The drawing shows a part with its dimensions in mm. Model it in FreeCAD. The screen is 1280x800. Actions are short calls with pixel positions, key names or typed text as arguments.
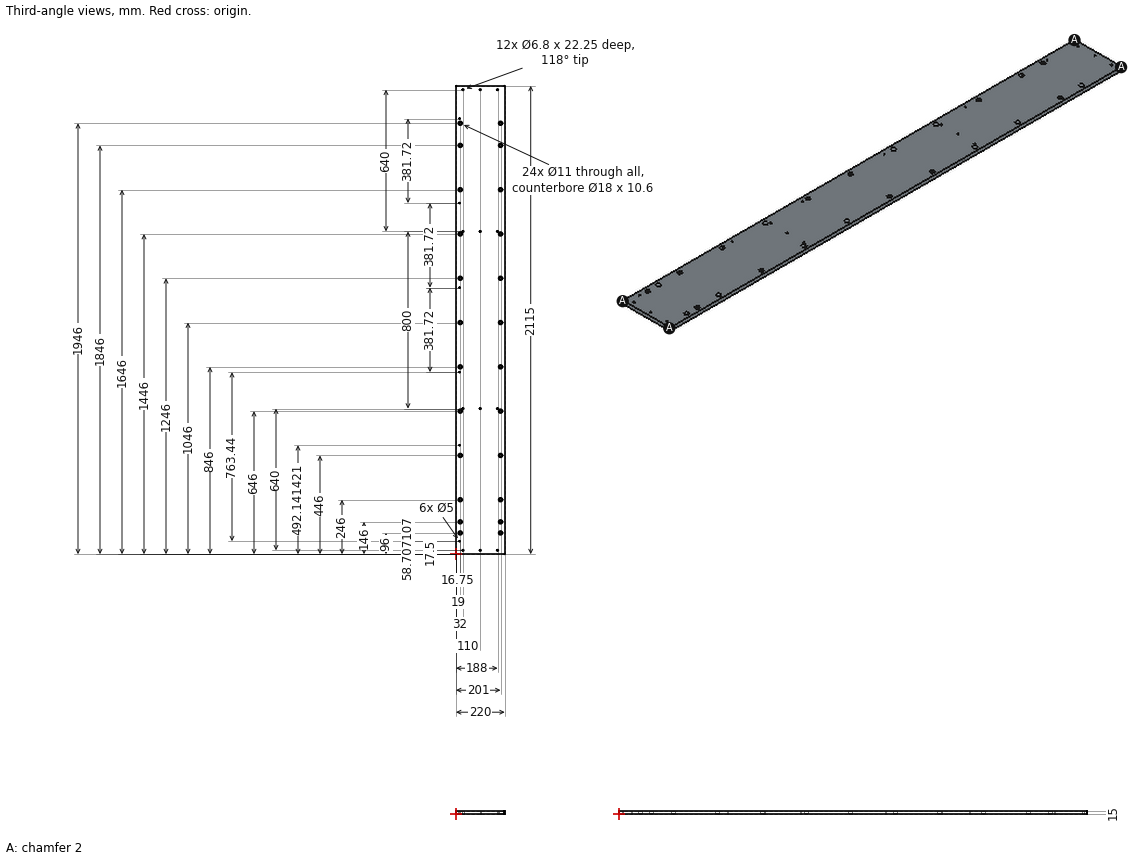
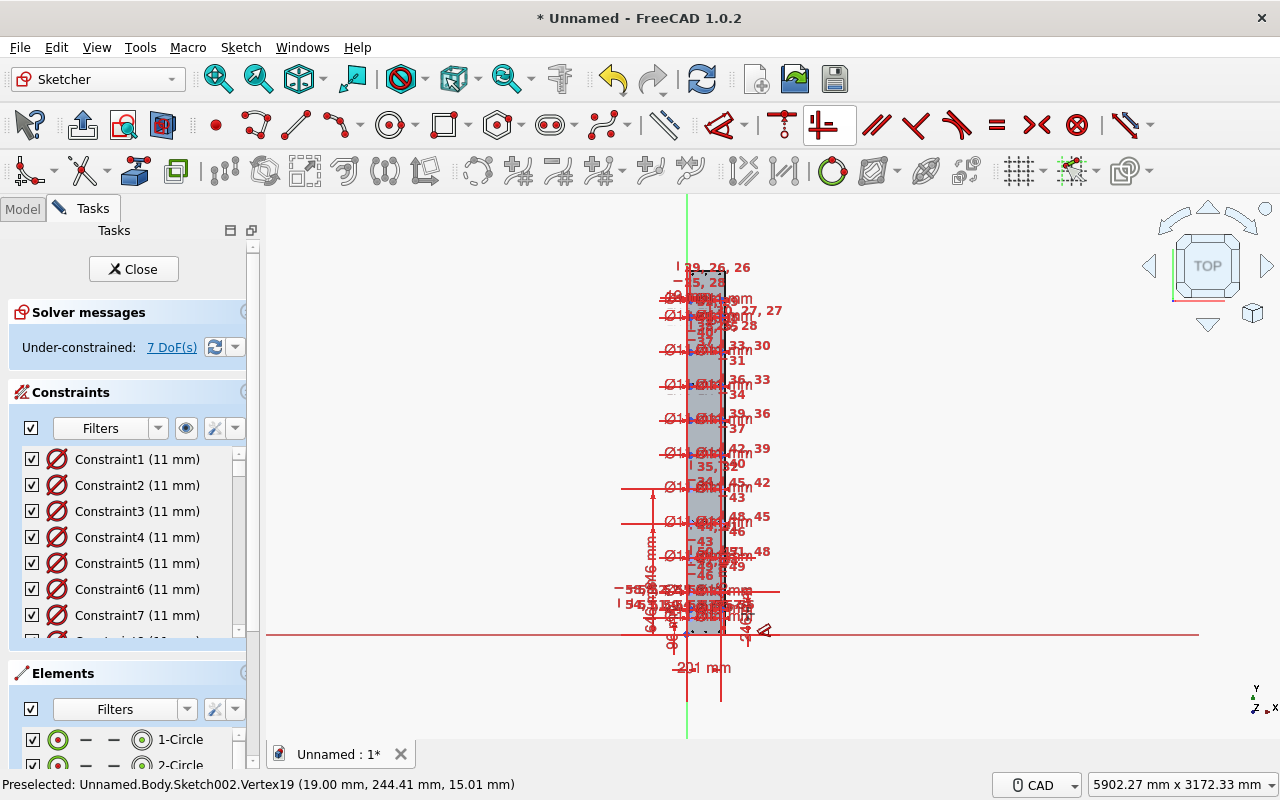
scroll(690, 610, up, 3)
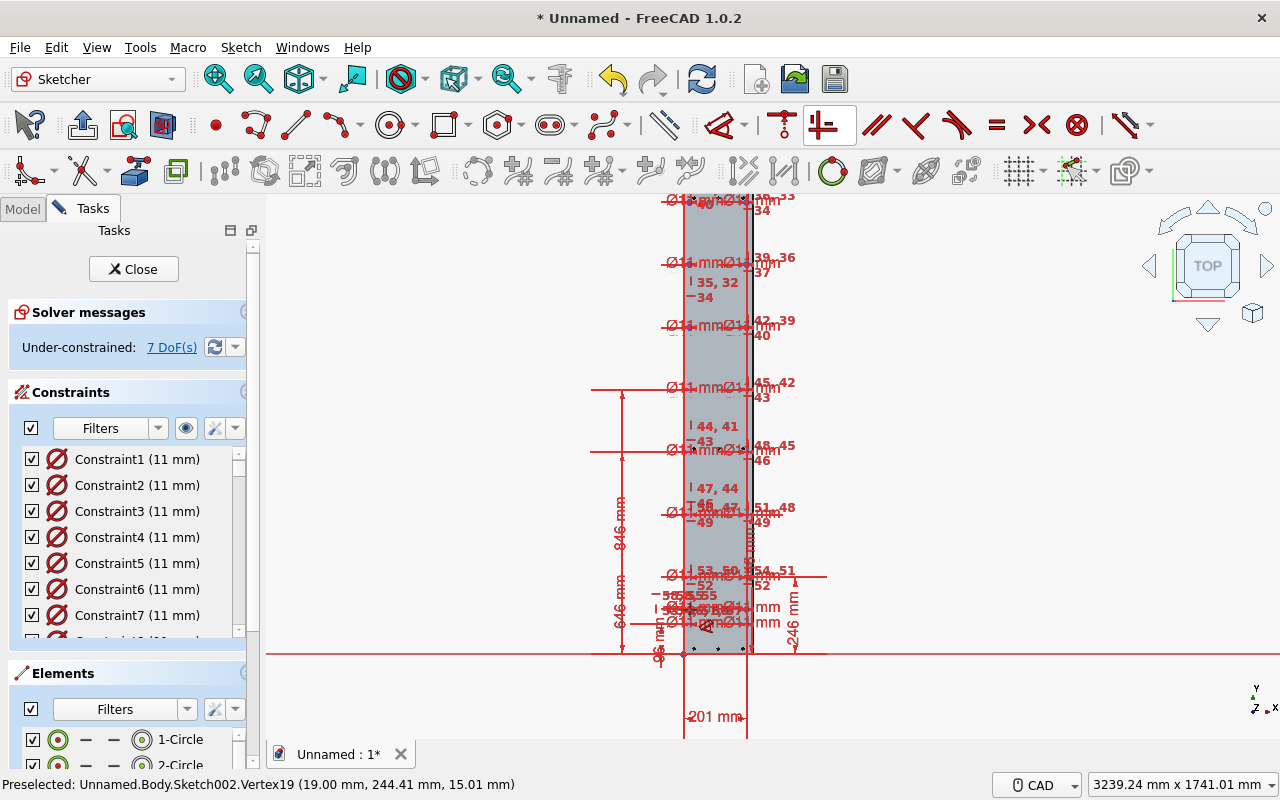
click(690, 609)
click(724, 616)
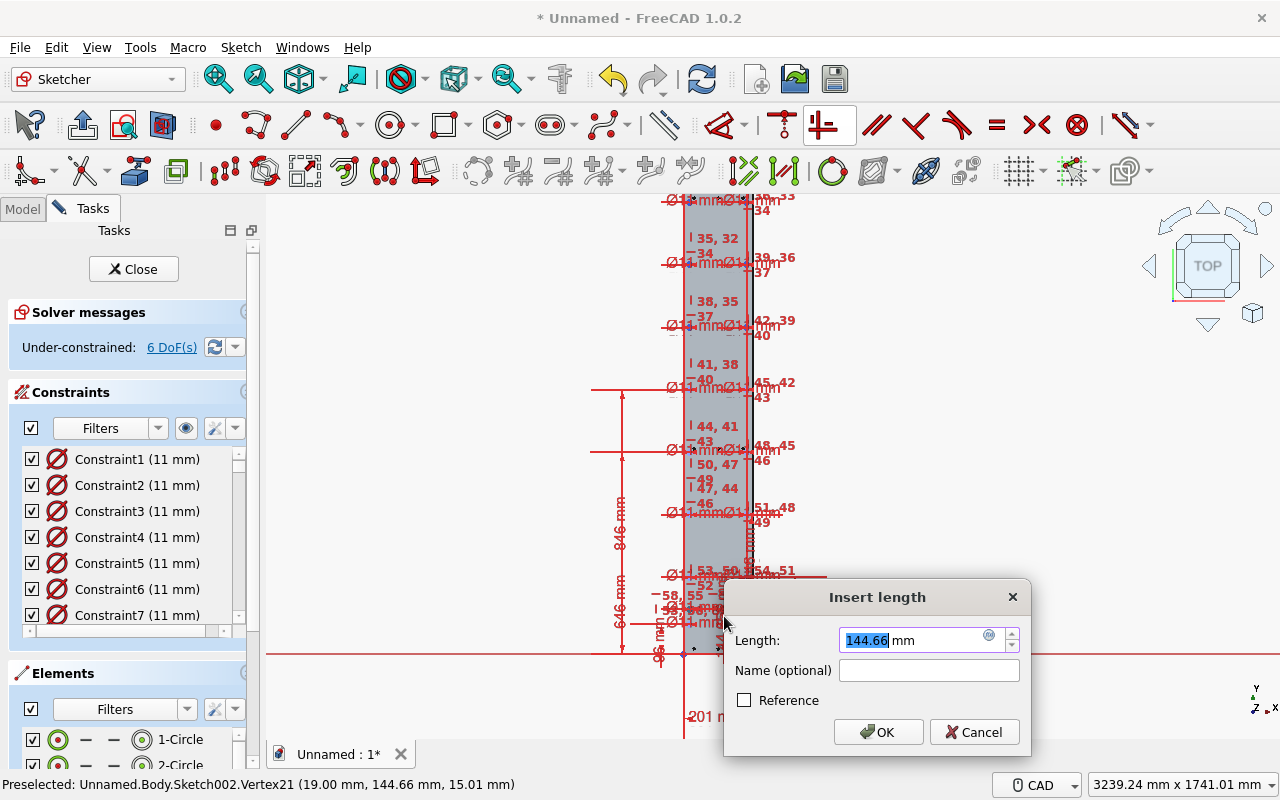
text(146)
key(Return)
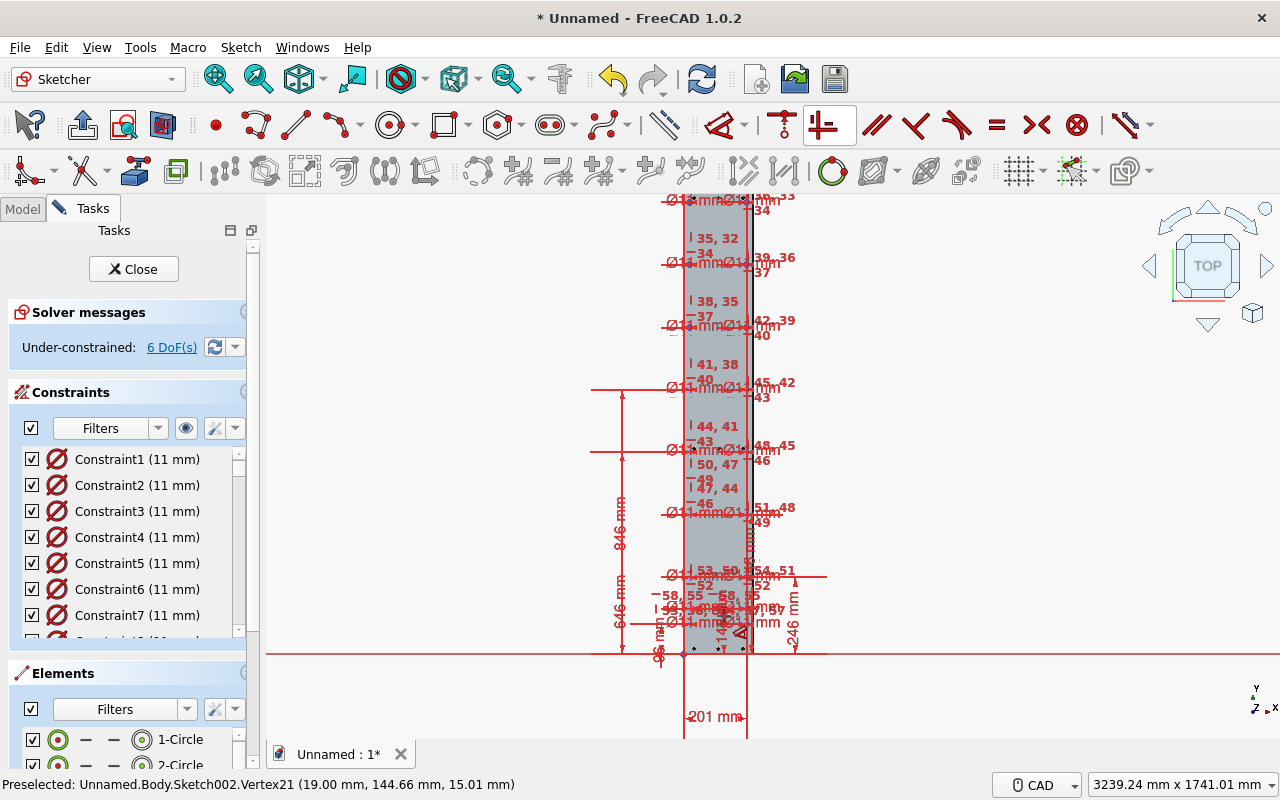
scroll(690, 609, down, 3)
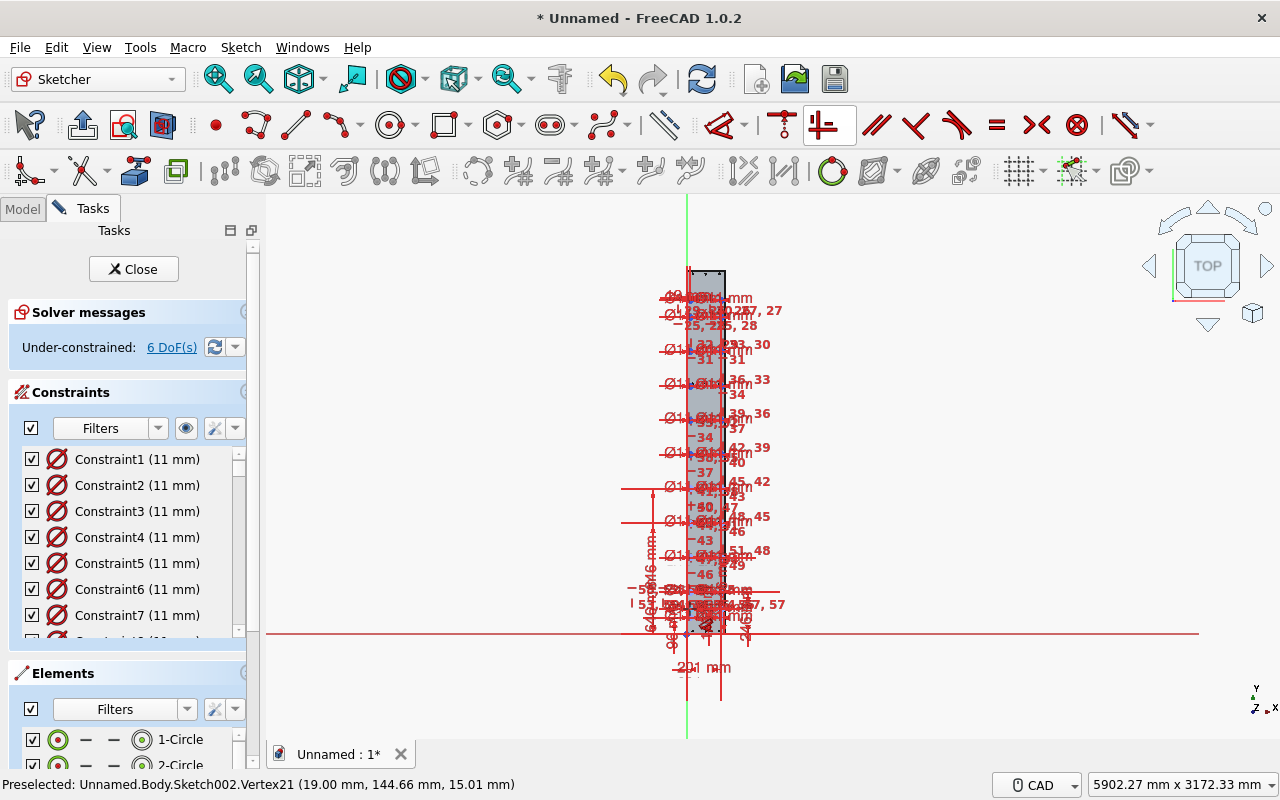
click(690, 300)
click(653, 467)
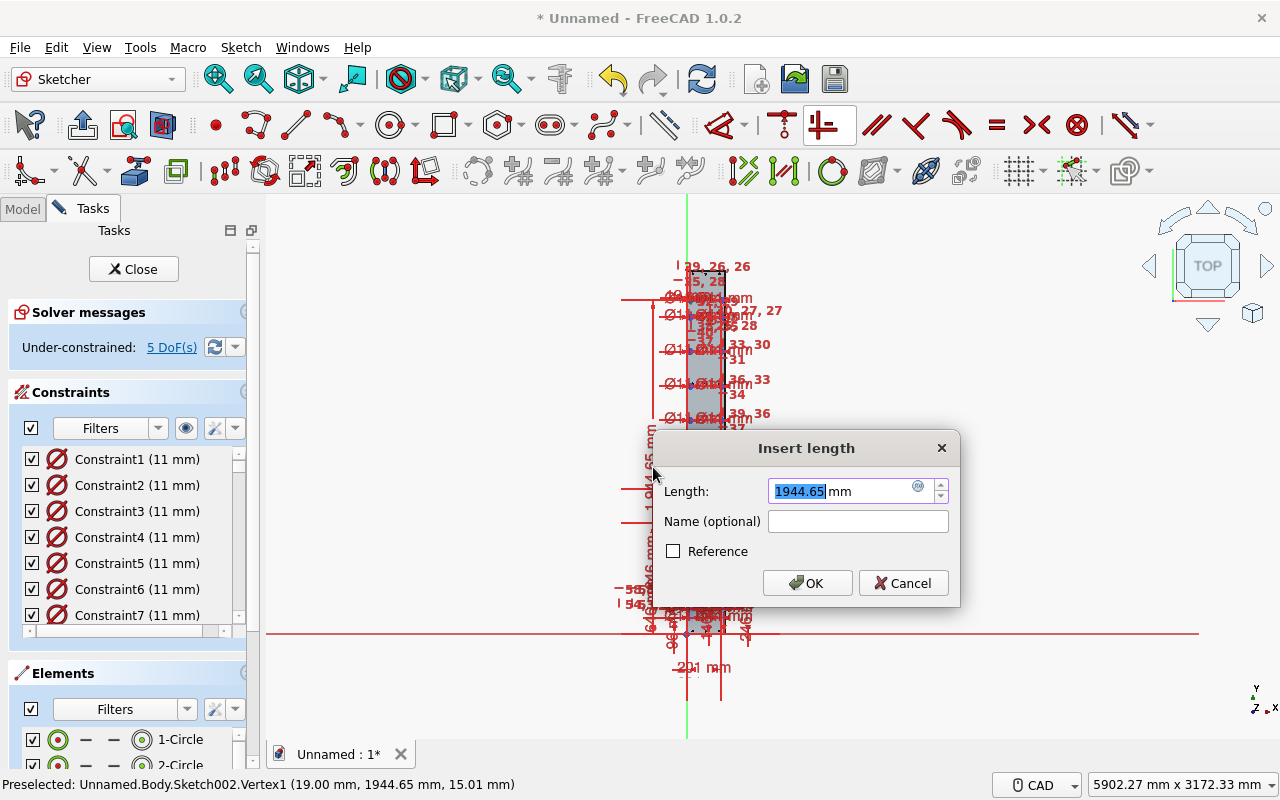
text(1946)
key(Return)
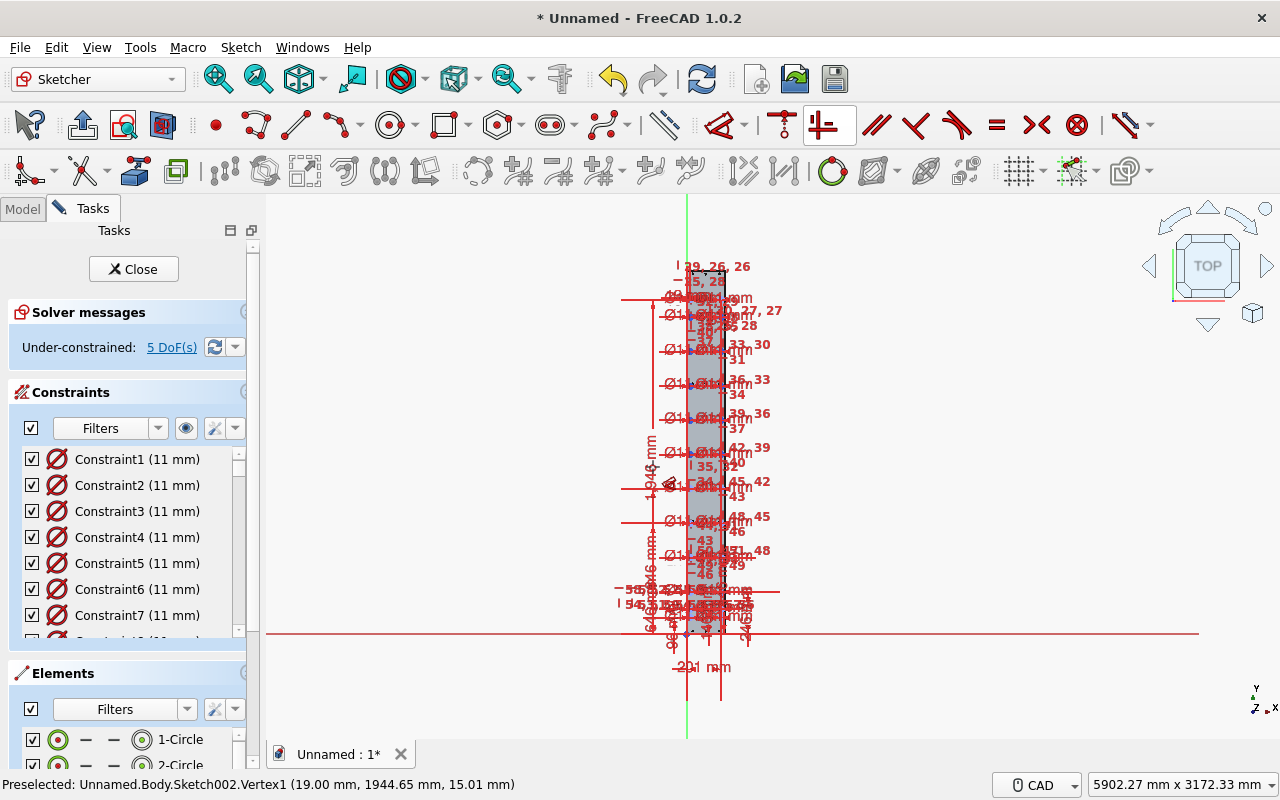
click(690, 317)
click(653, 403)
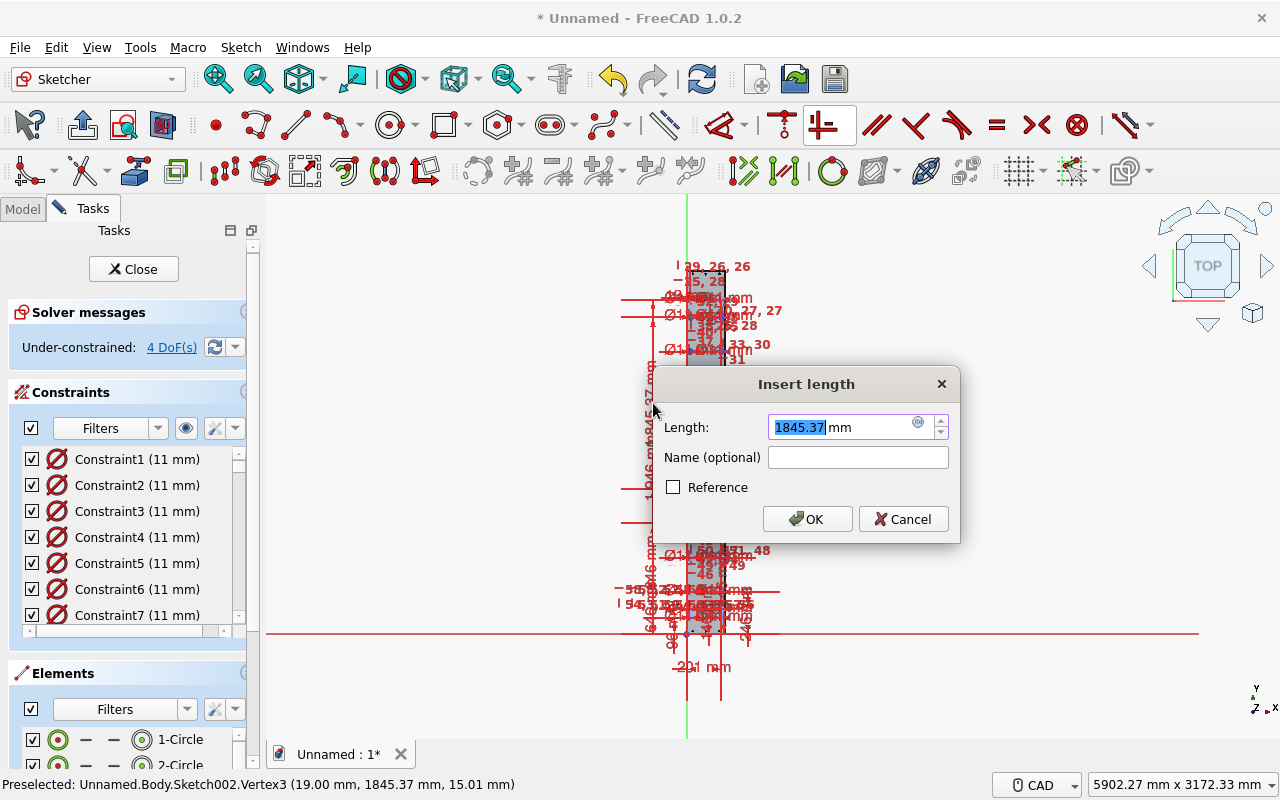
text(1846)
key(Return)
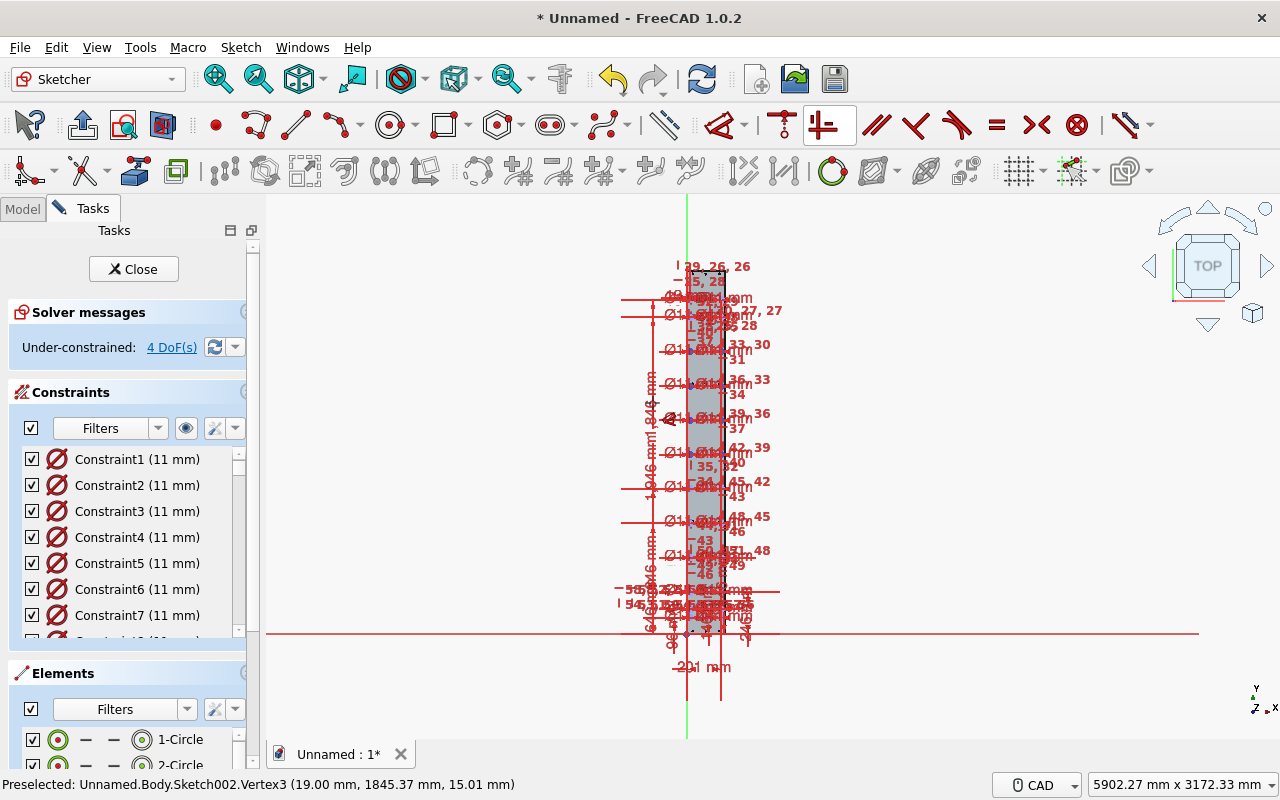
click(690, 352)
click(653, 493)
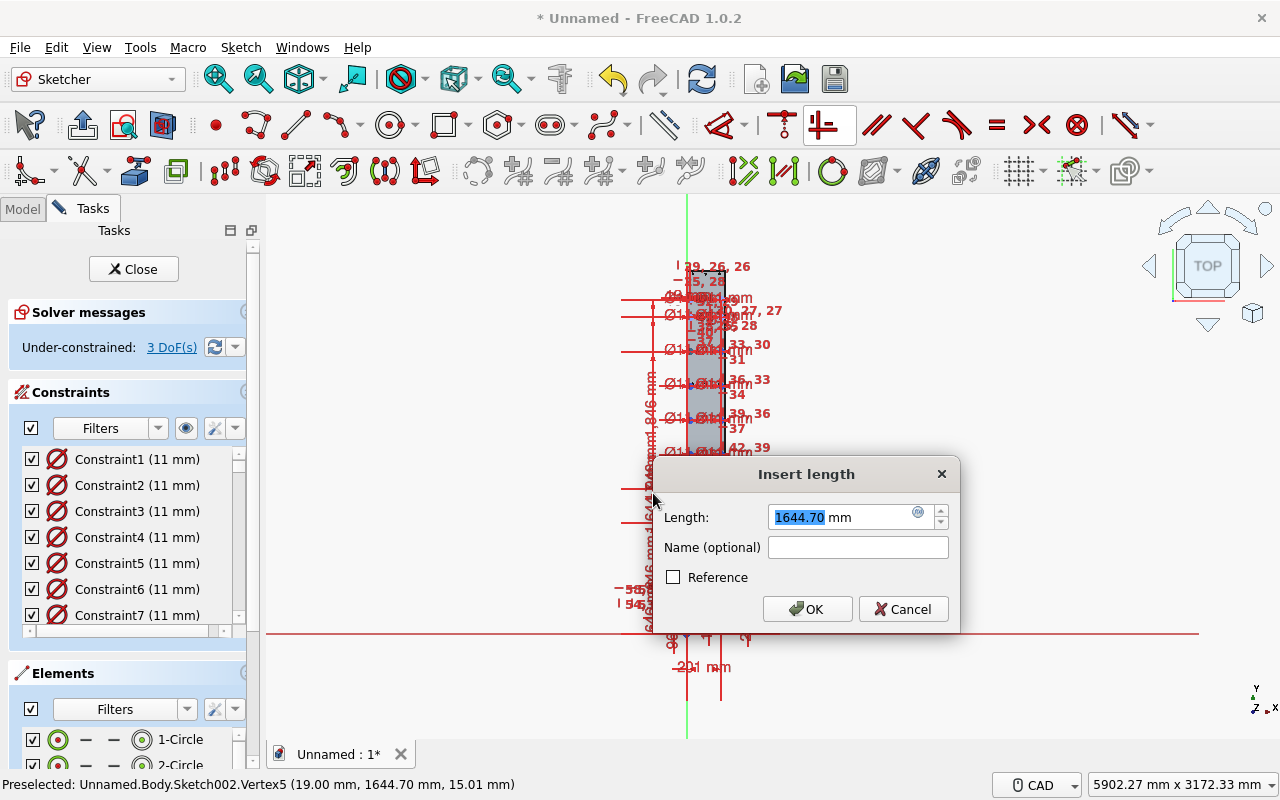
text(1646)
key(Return)